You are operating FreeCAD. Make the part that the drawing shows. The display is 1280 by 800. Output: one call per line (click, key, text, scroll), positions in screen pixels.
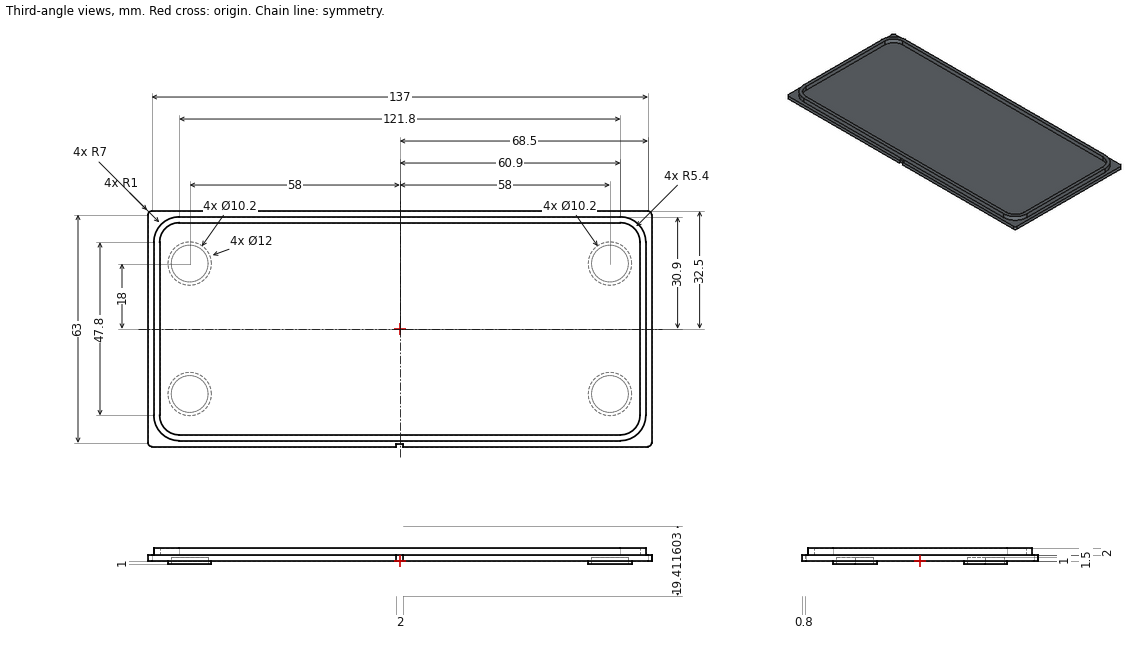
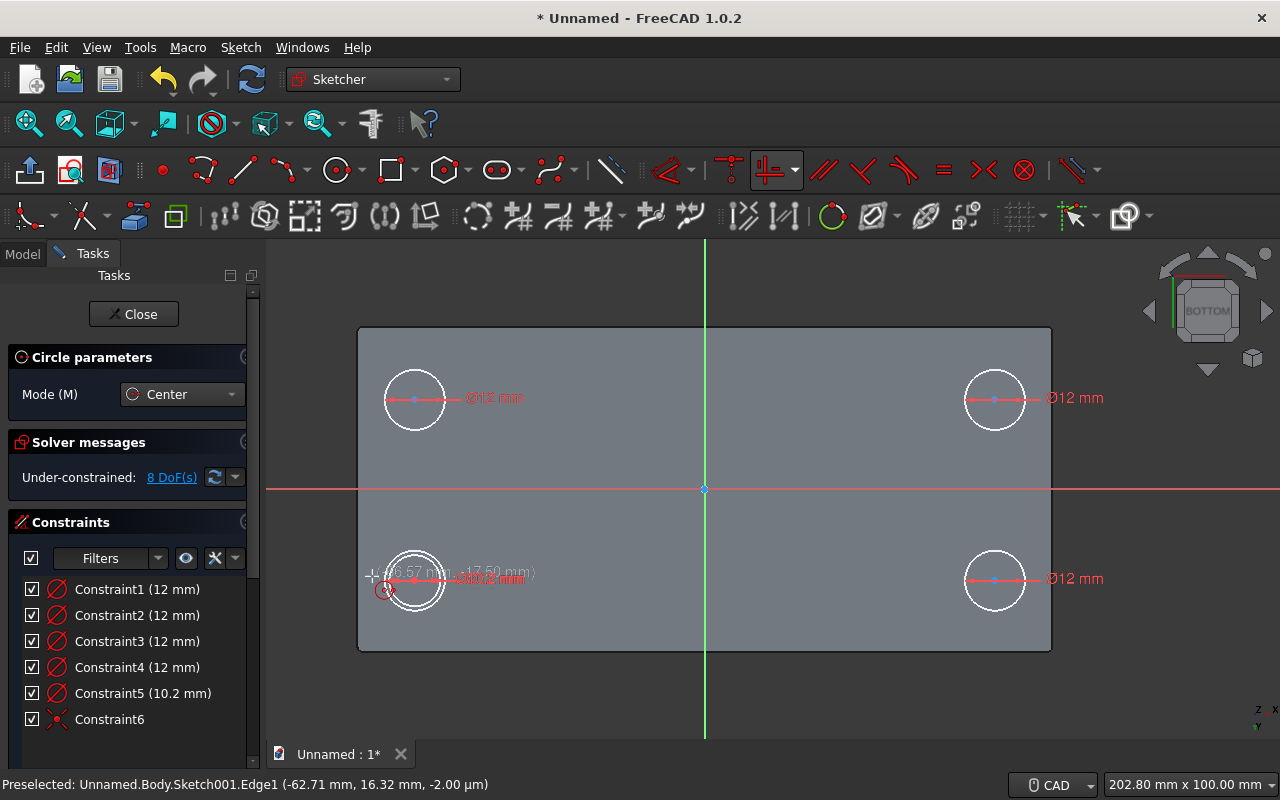
click(995, 581)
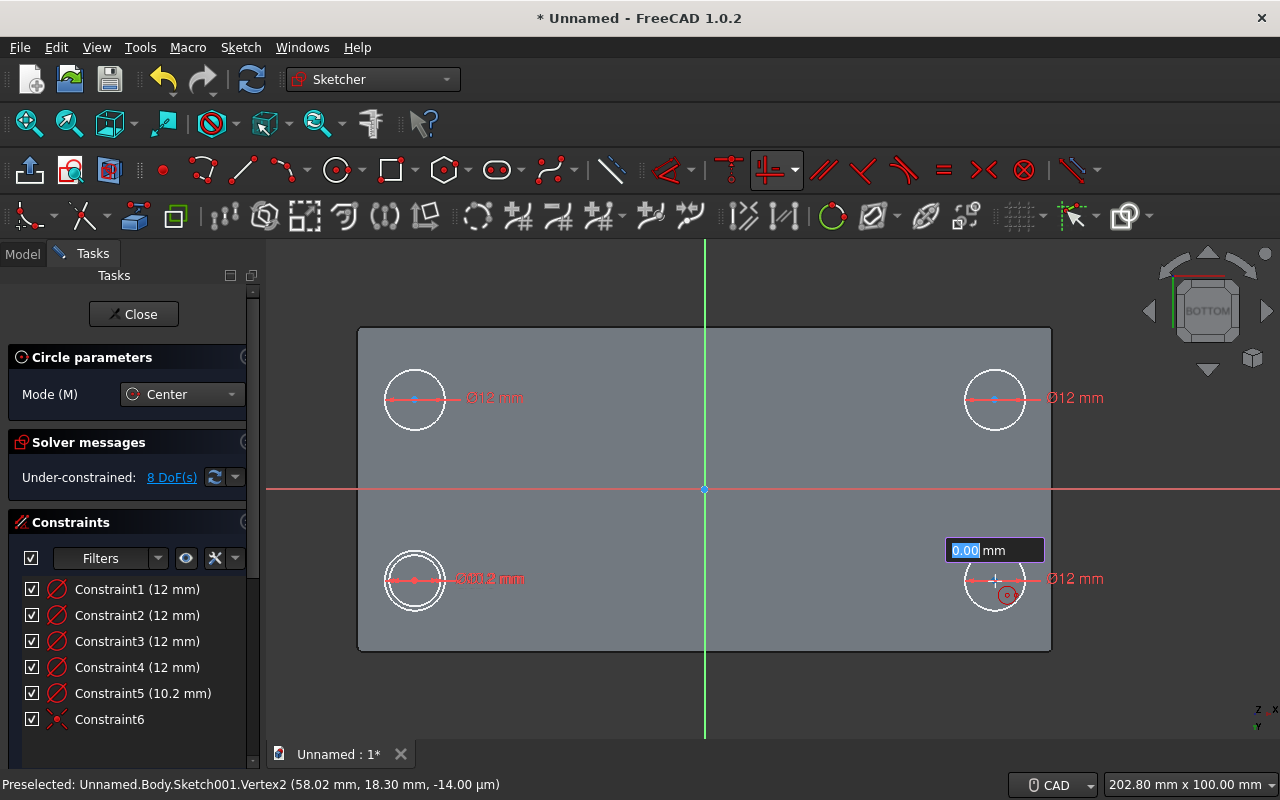
scroll(971, 571, up, 7)
move(969, 567)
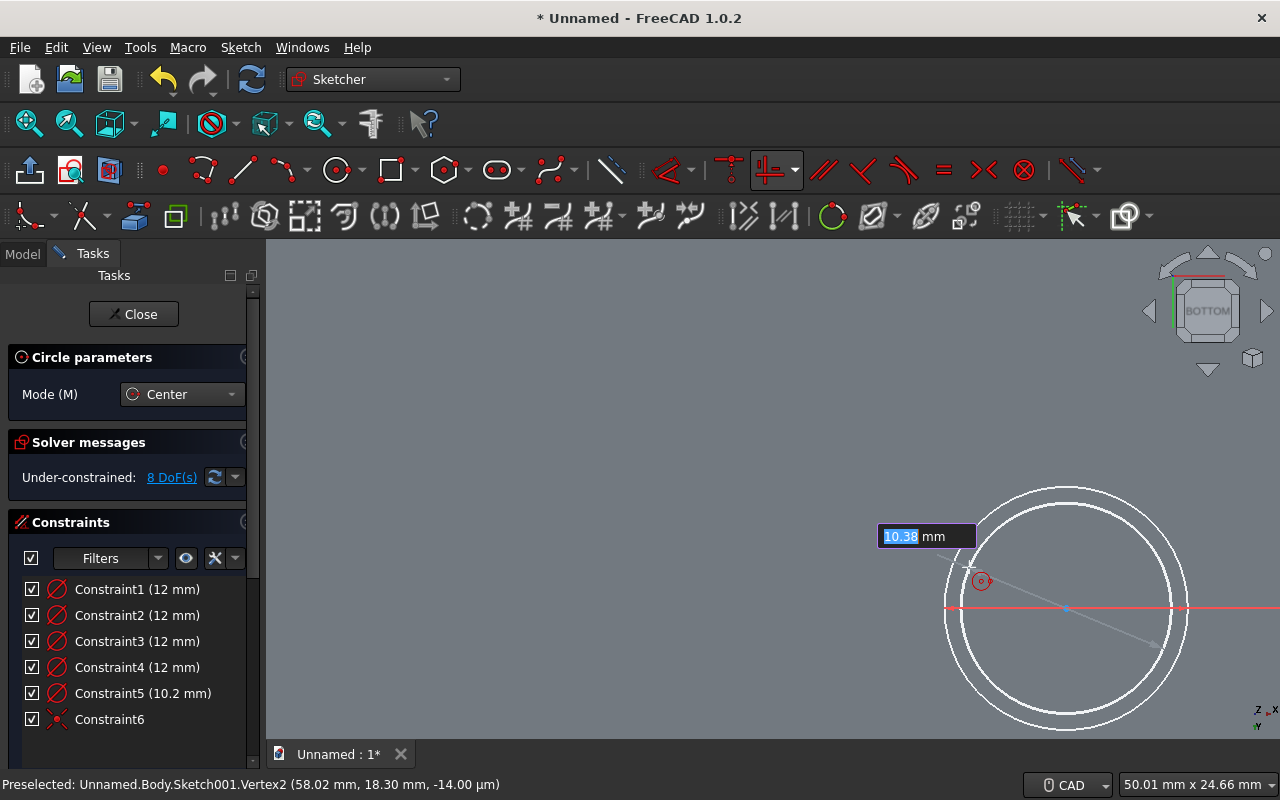
text(10.2)
key(Return)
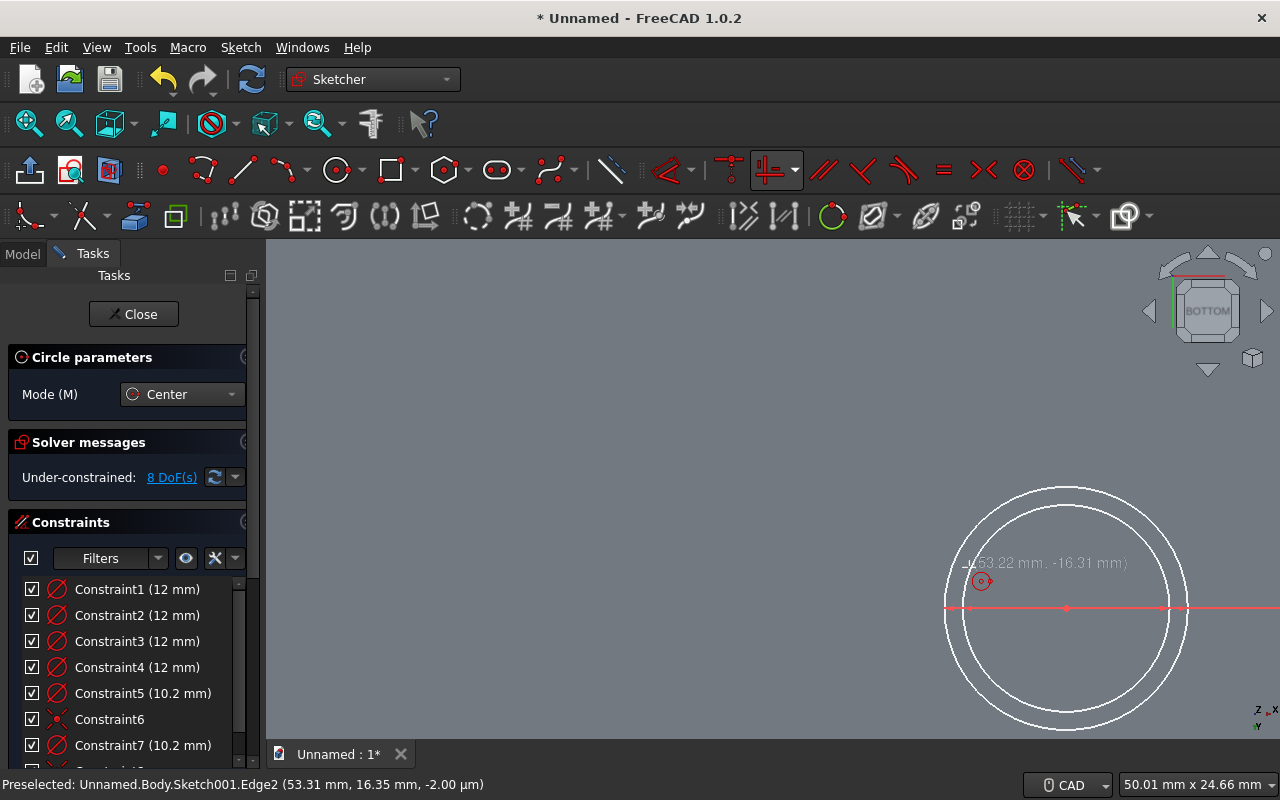
scroll(971, 571, down, 7)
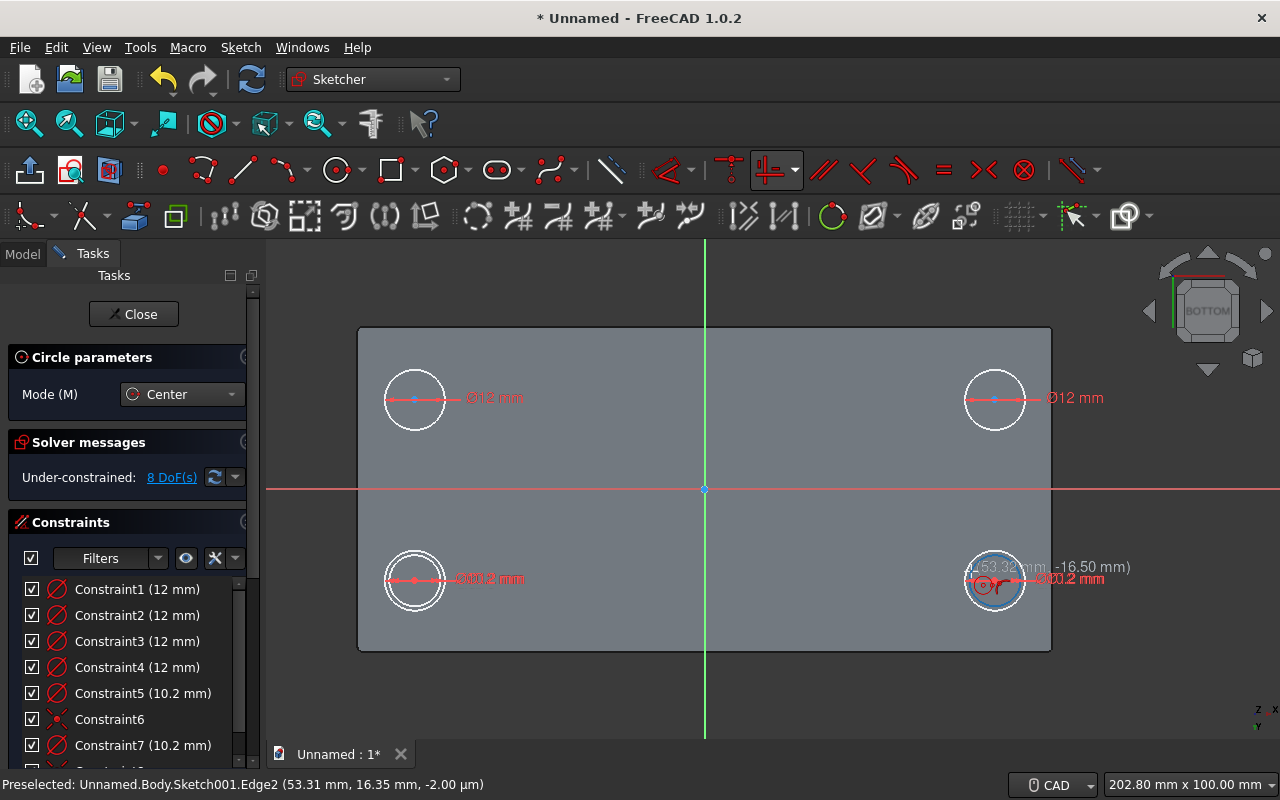
click(415, 400)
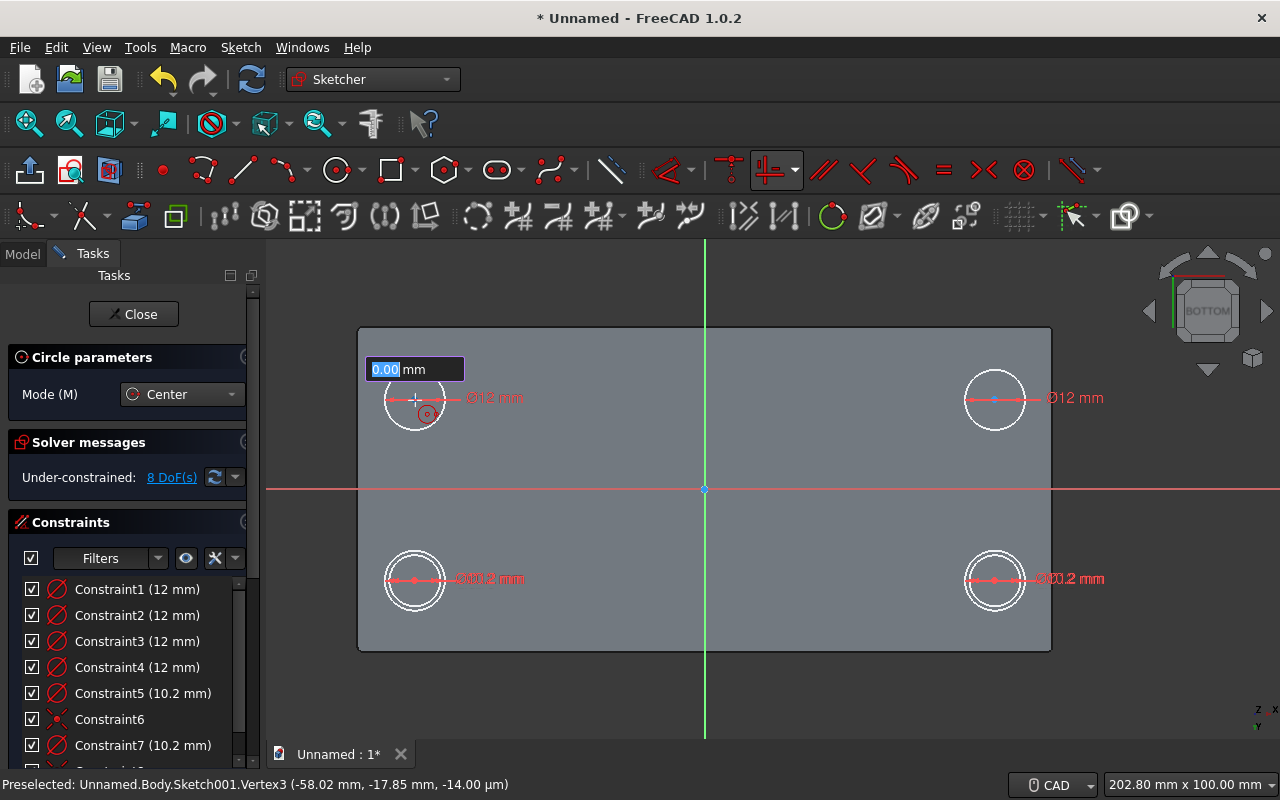
scroll(391, 391, up, 7)
move(390, 388)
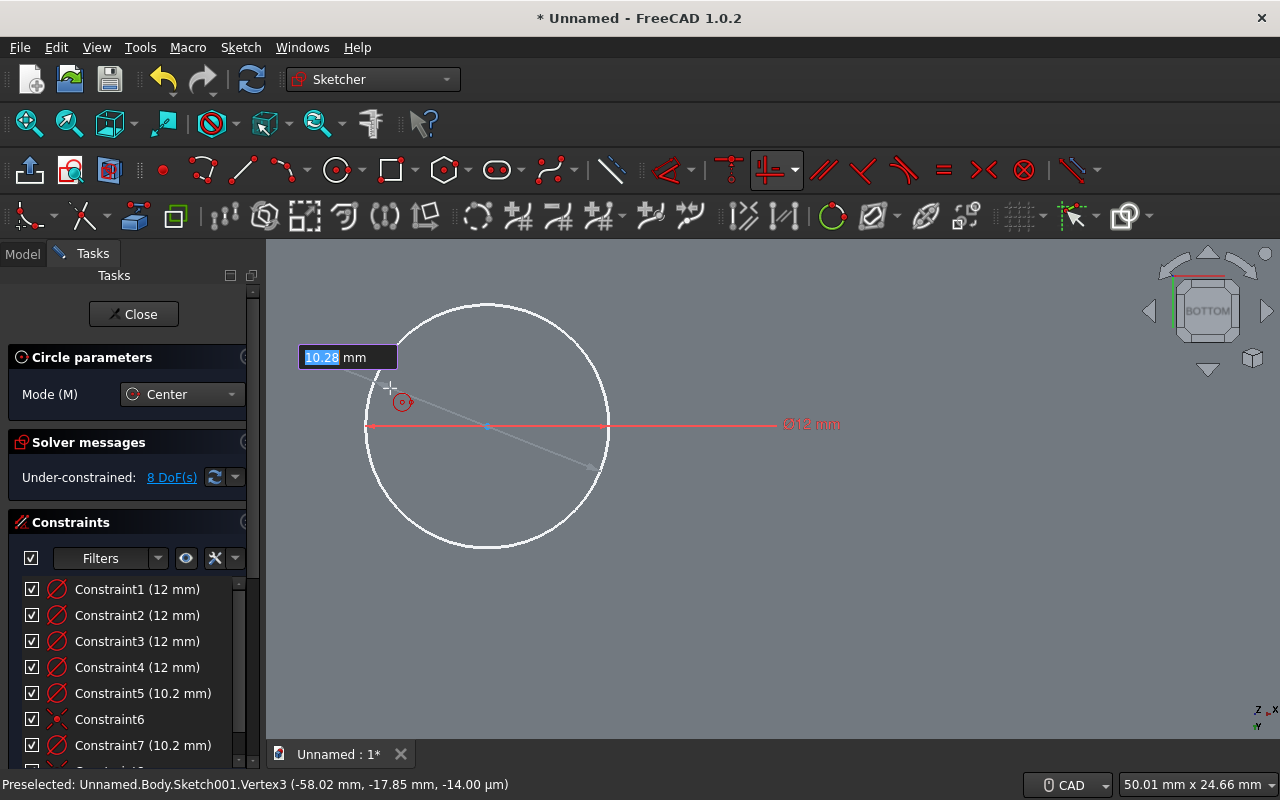
text(10.2)
key(Return)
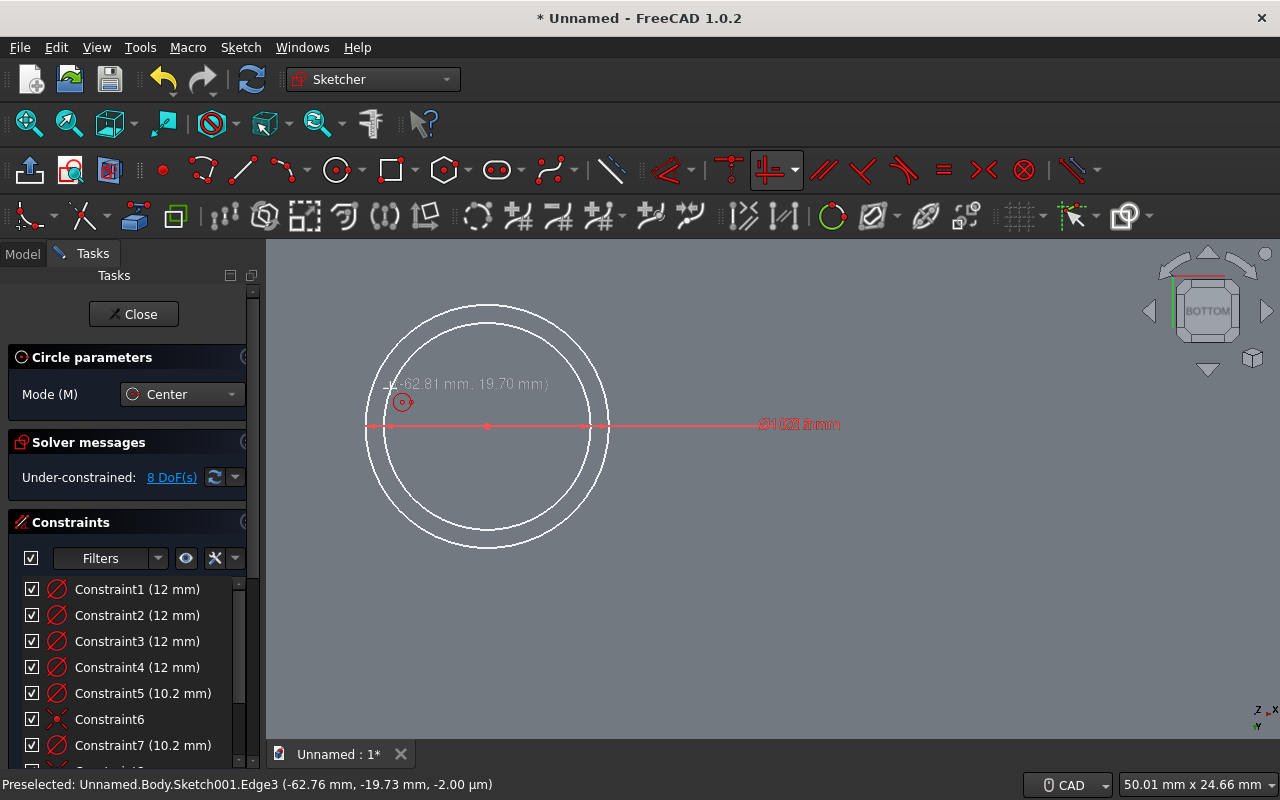
scroll(391, 391, down, 7)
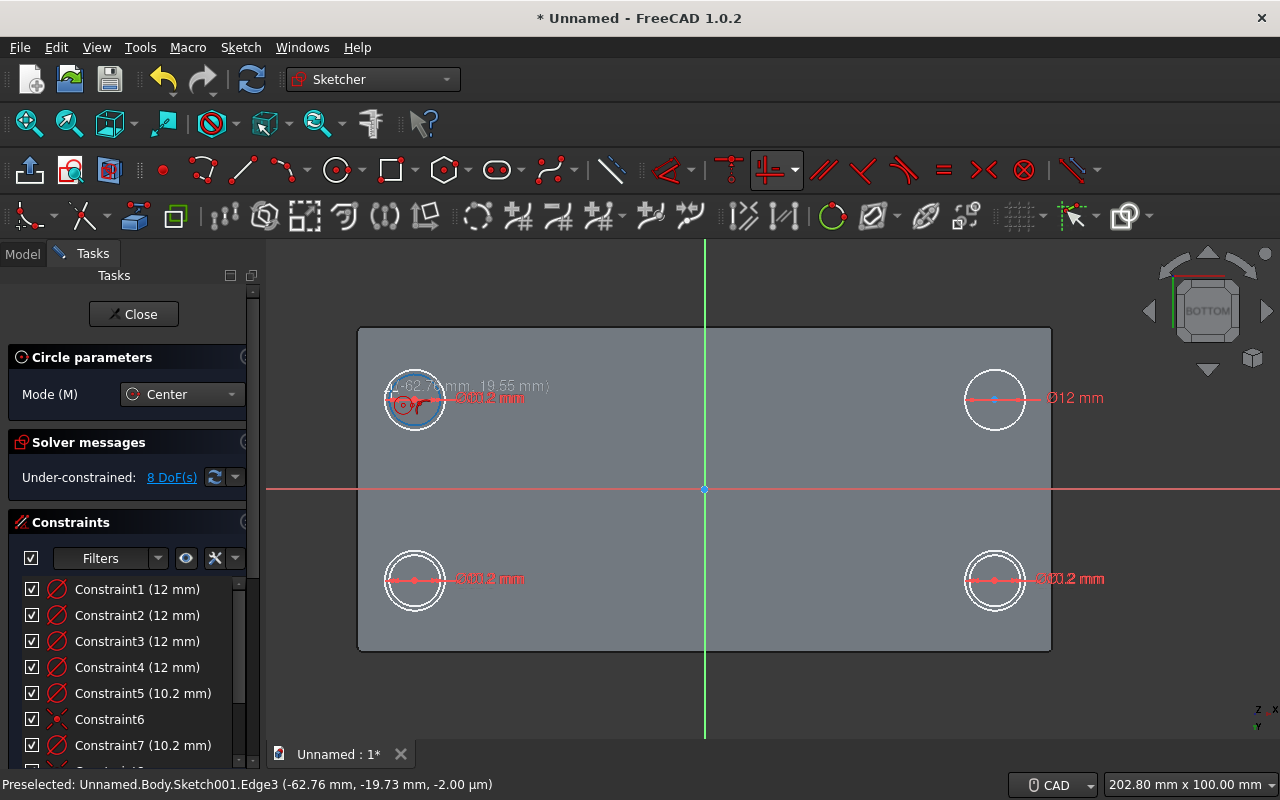
click(995, 400)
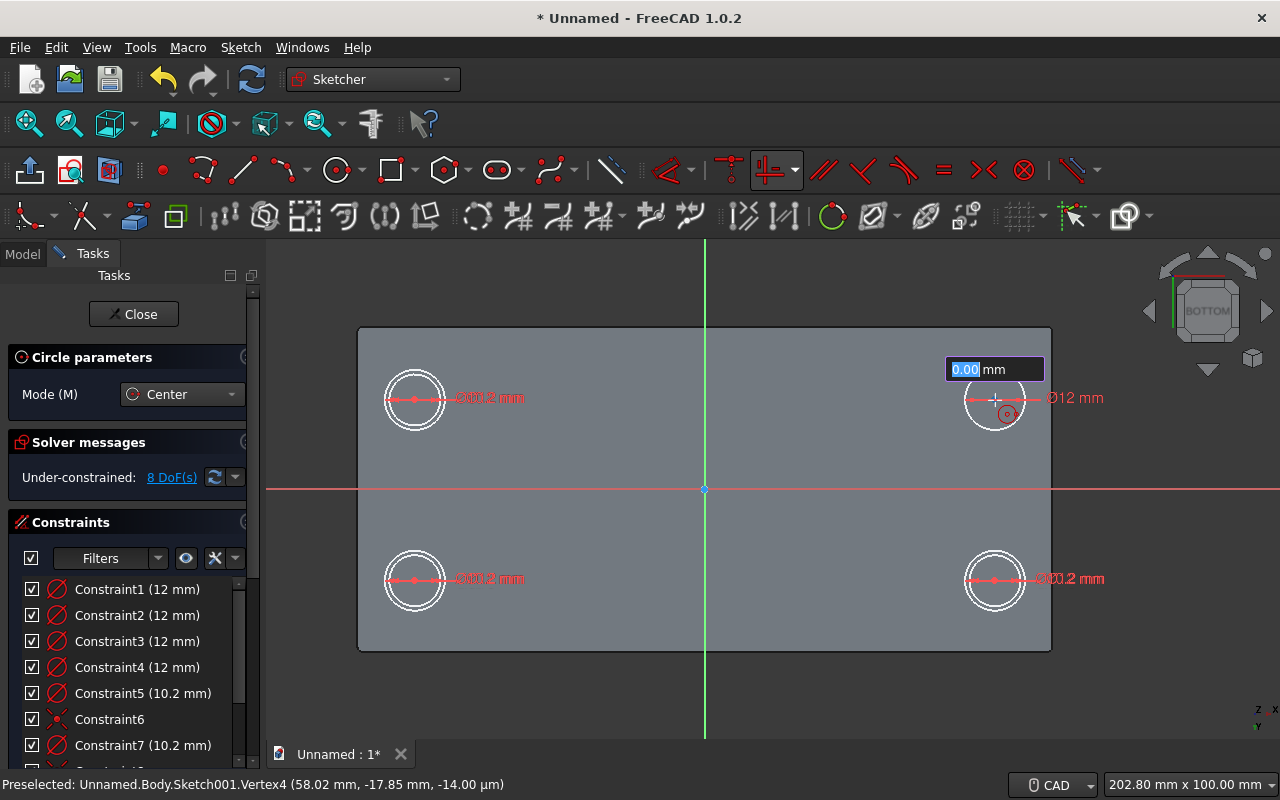
scroll(971, 391, up, 7)
move(969, 388)